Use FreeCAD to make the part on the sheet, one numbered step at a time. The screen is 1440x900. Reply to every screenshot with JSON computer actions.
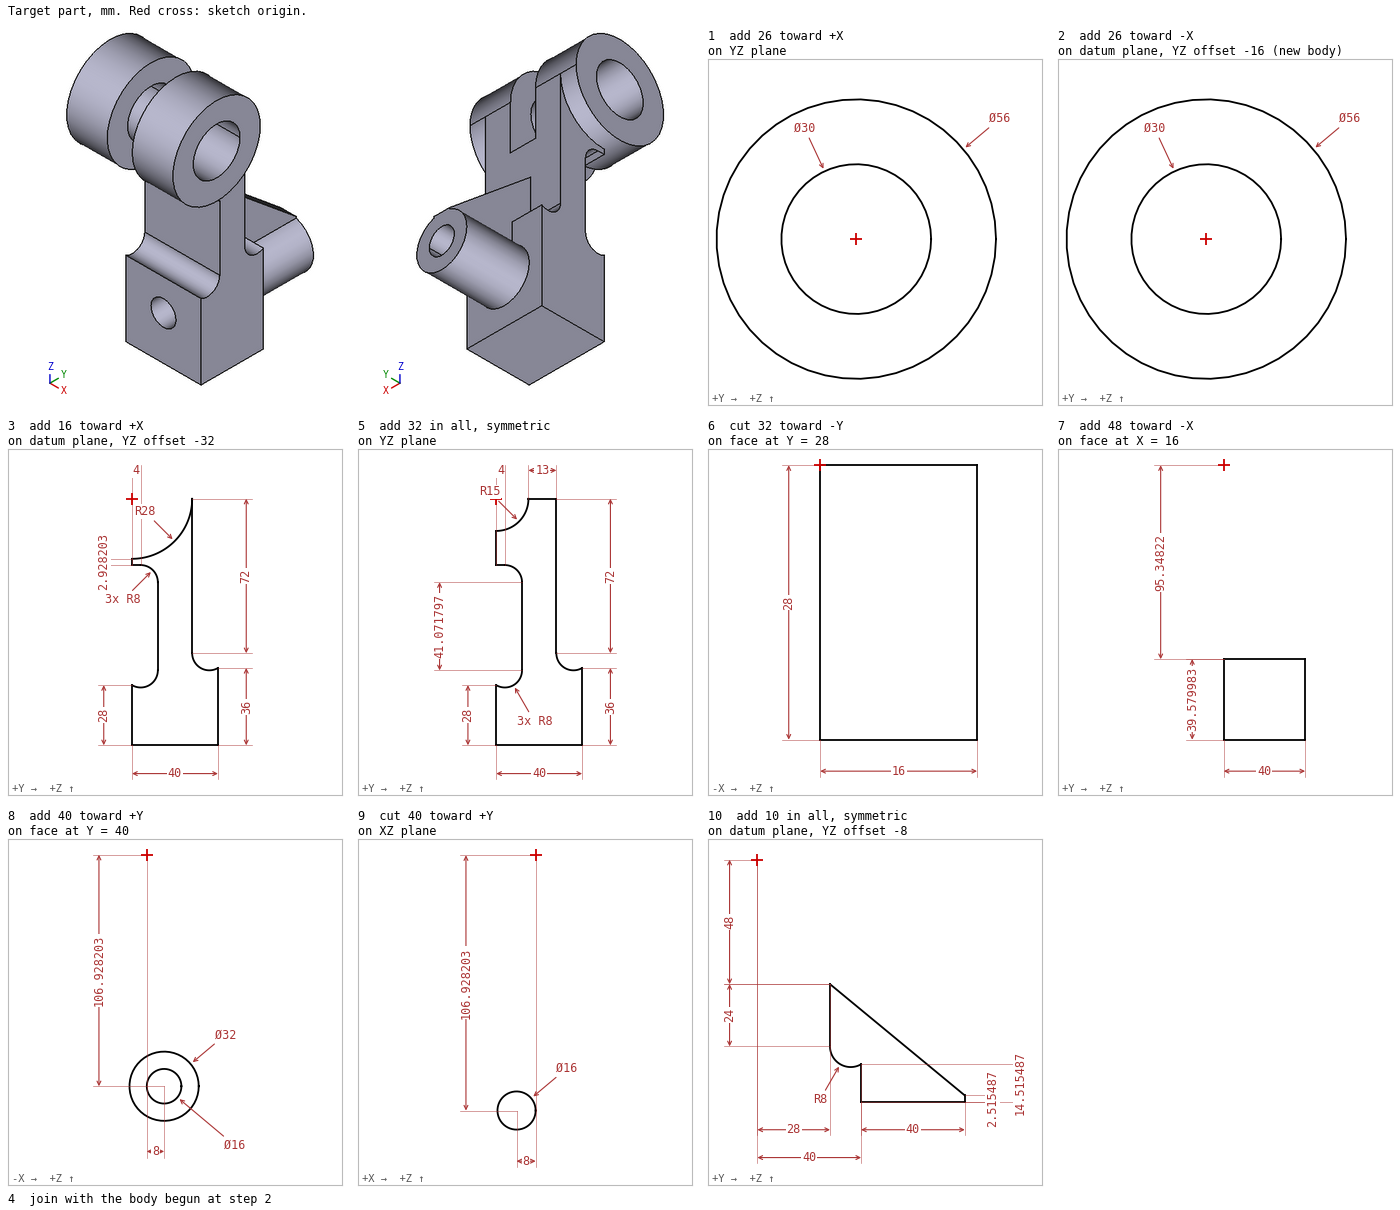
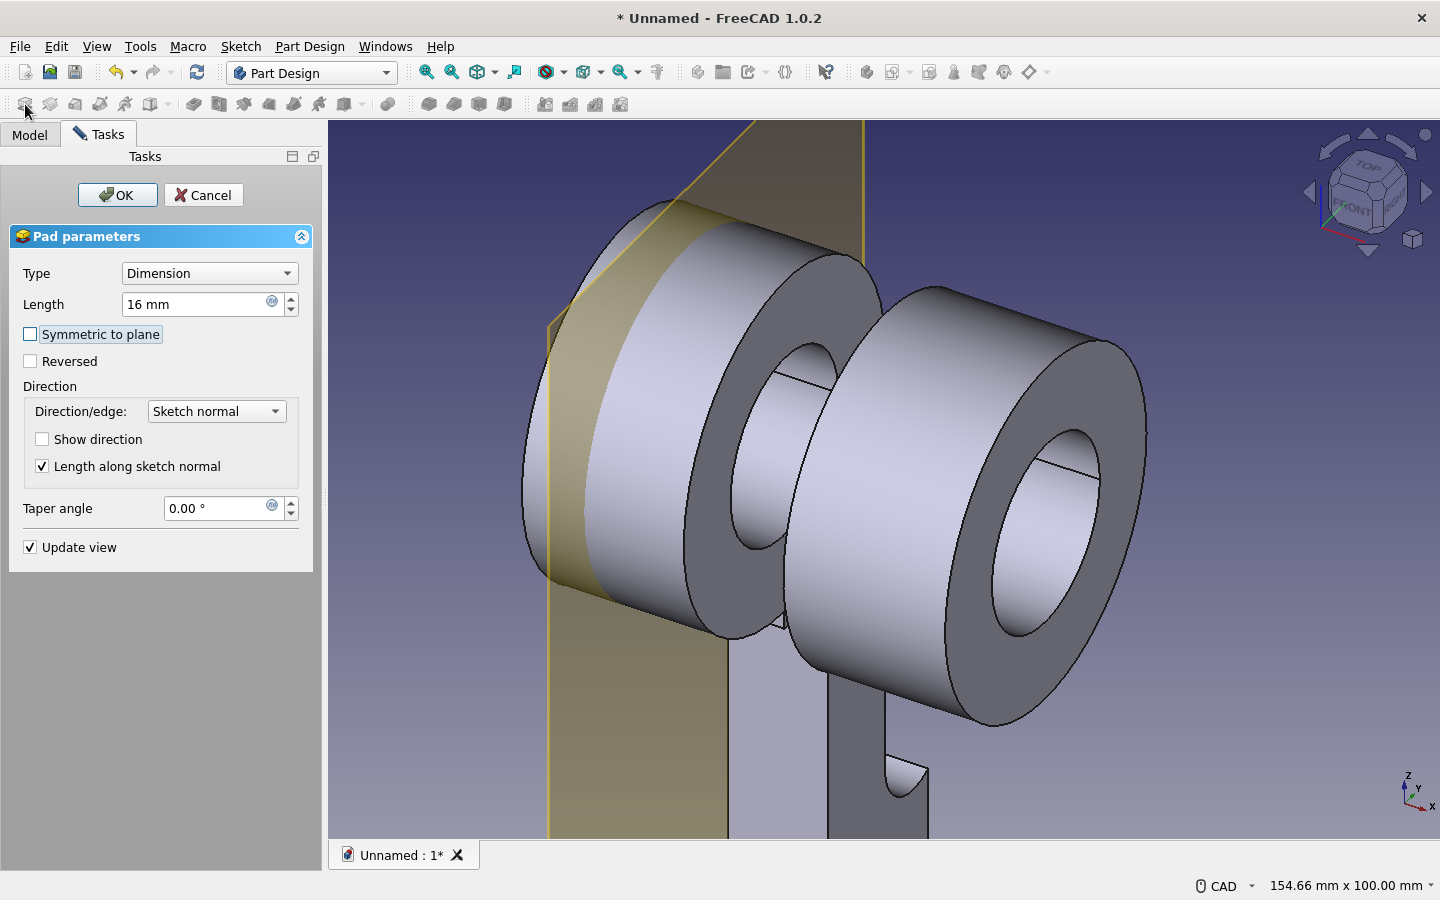
{"action": "left_click", "coordinate": [118, 195]}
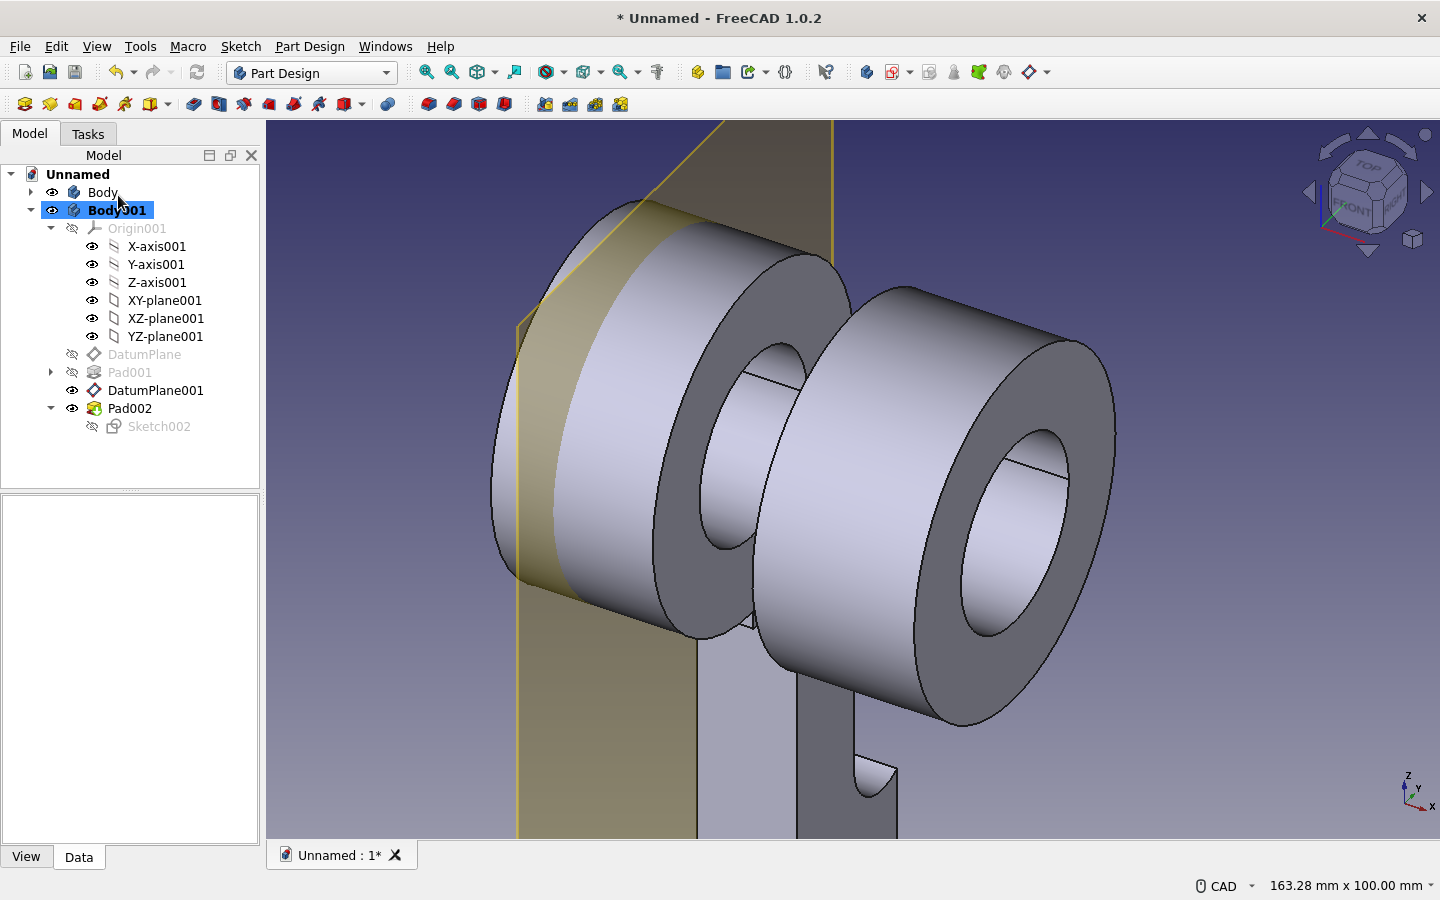
{"action": "left_click", "coordinate": [117, 390]}
{"action": "key", "text": "space"}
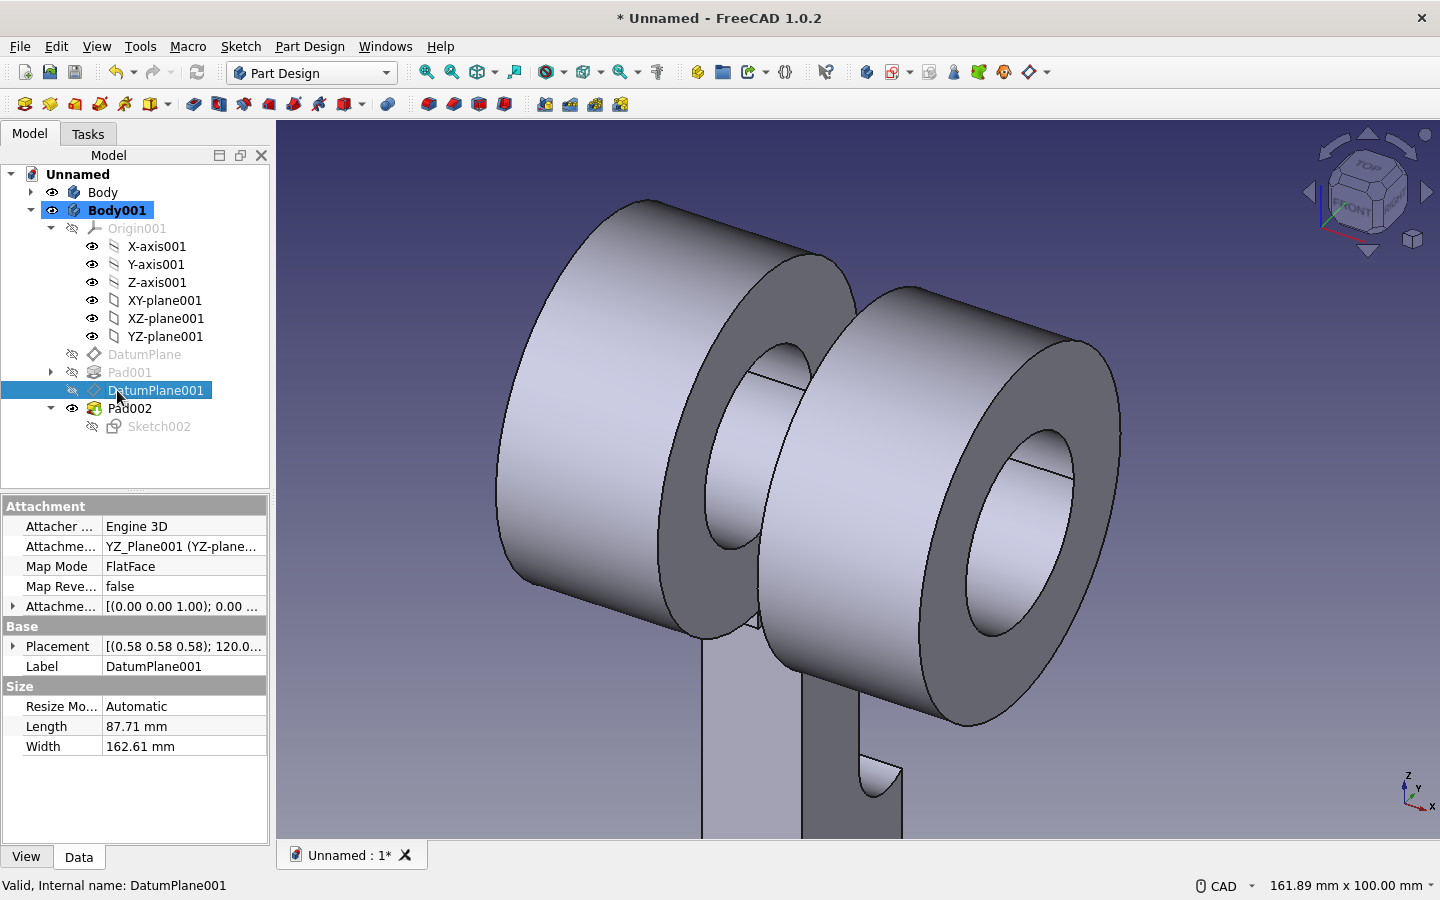
{"action": "key", "text": "v f"}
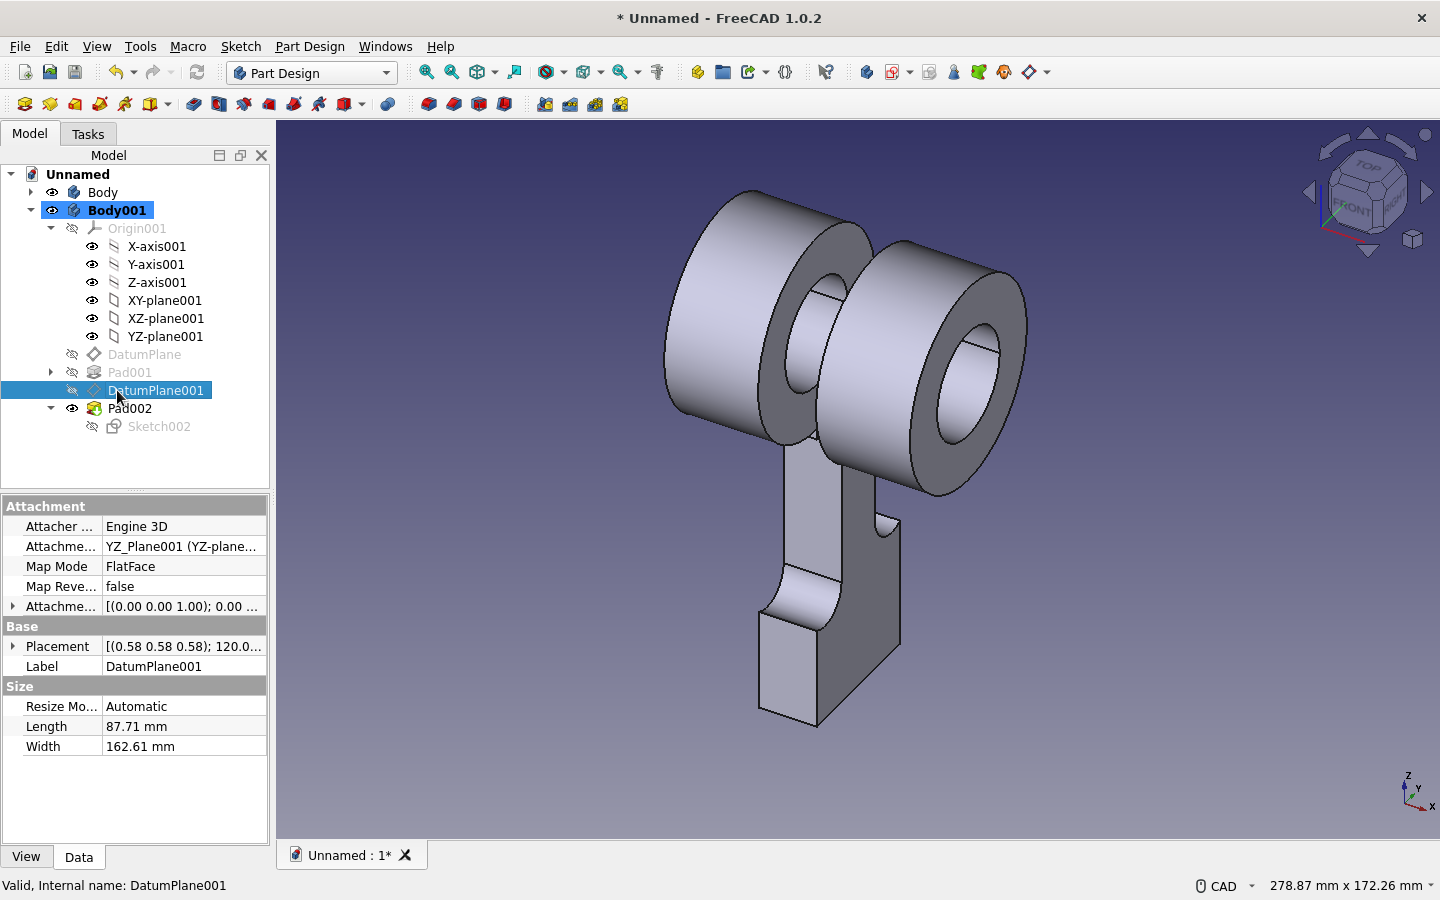
{"action": "double_click", "coordinate": [97, 192]}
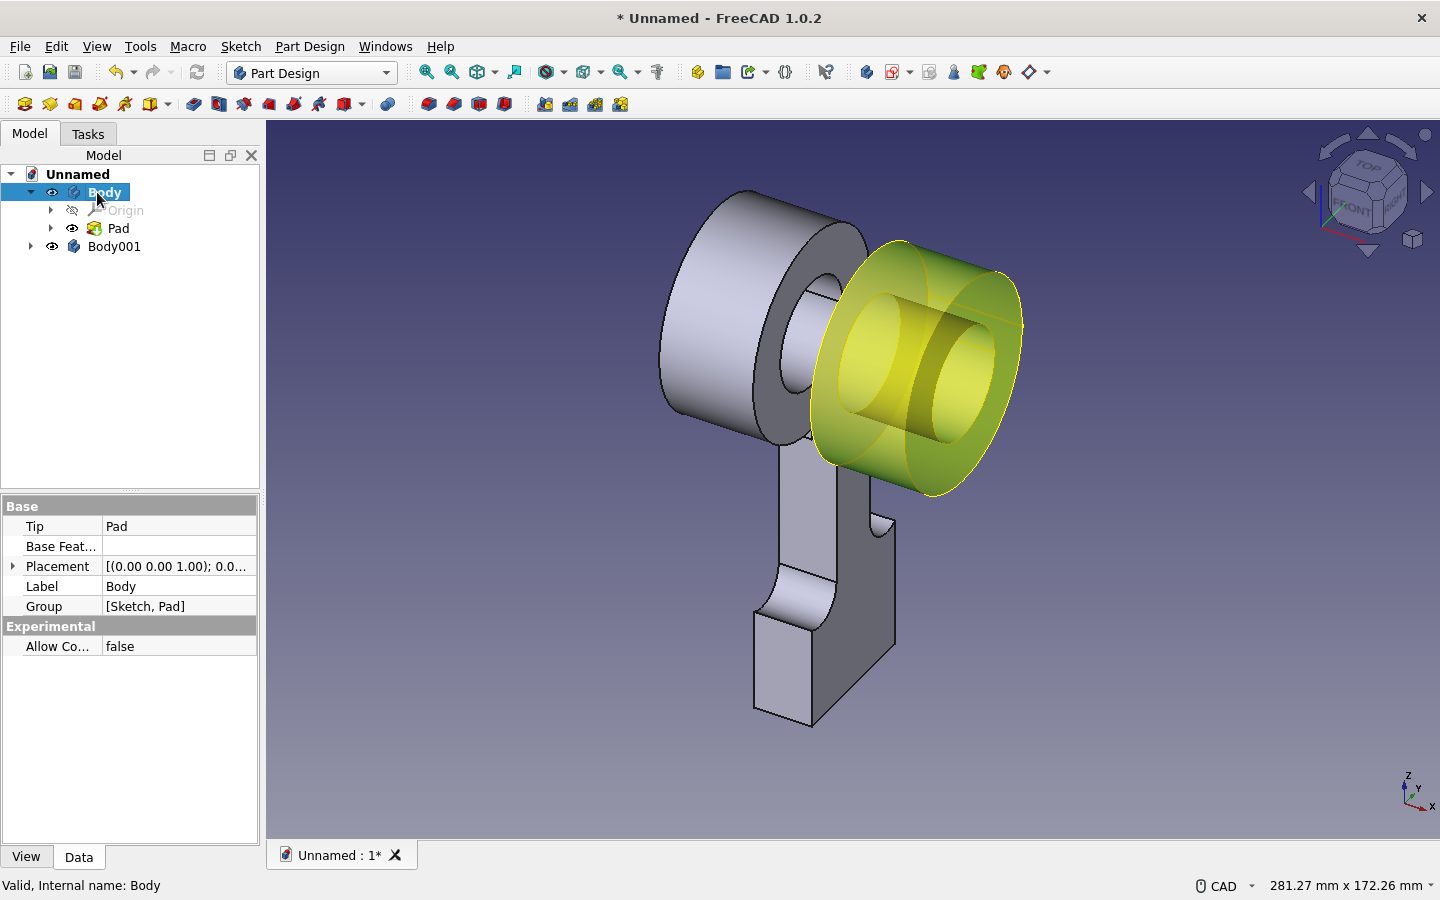
{"action": "left_click", "coordinate": [97, 192]}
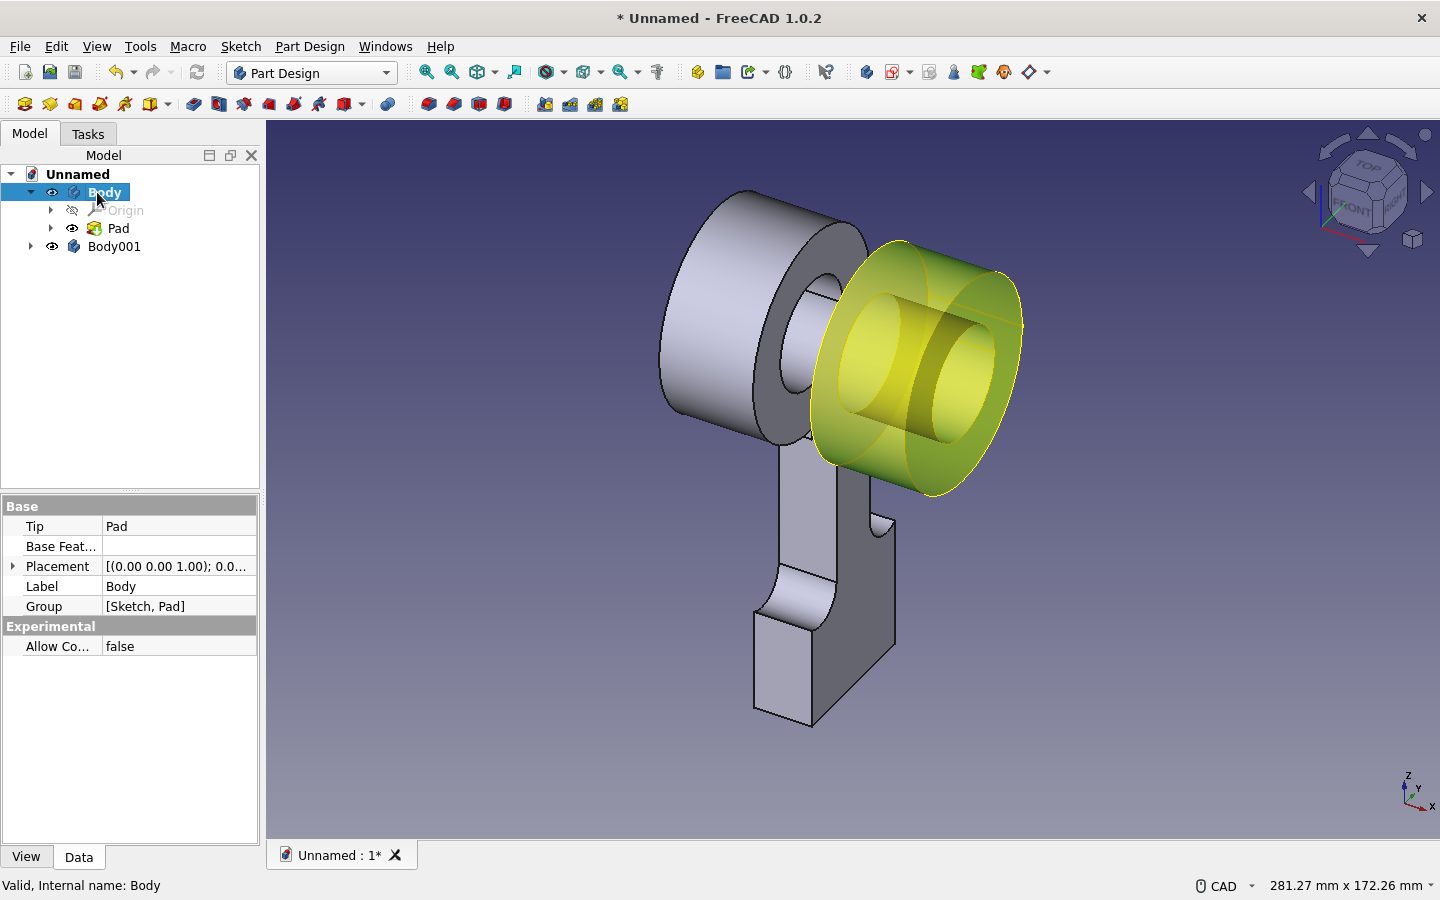
{"action": "left_click", "coordinate": [148, 646]}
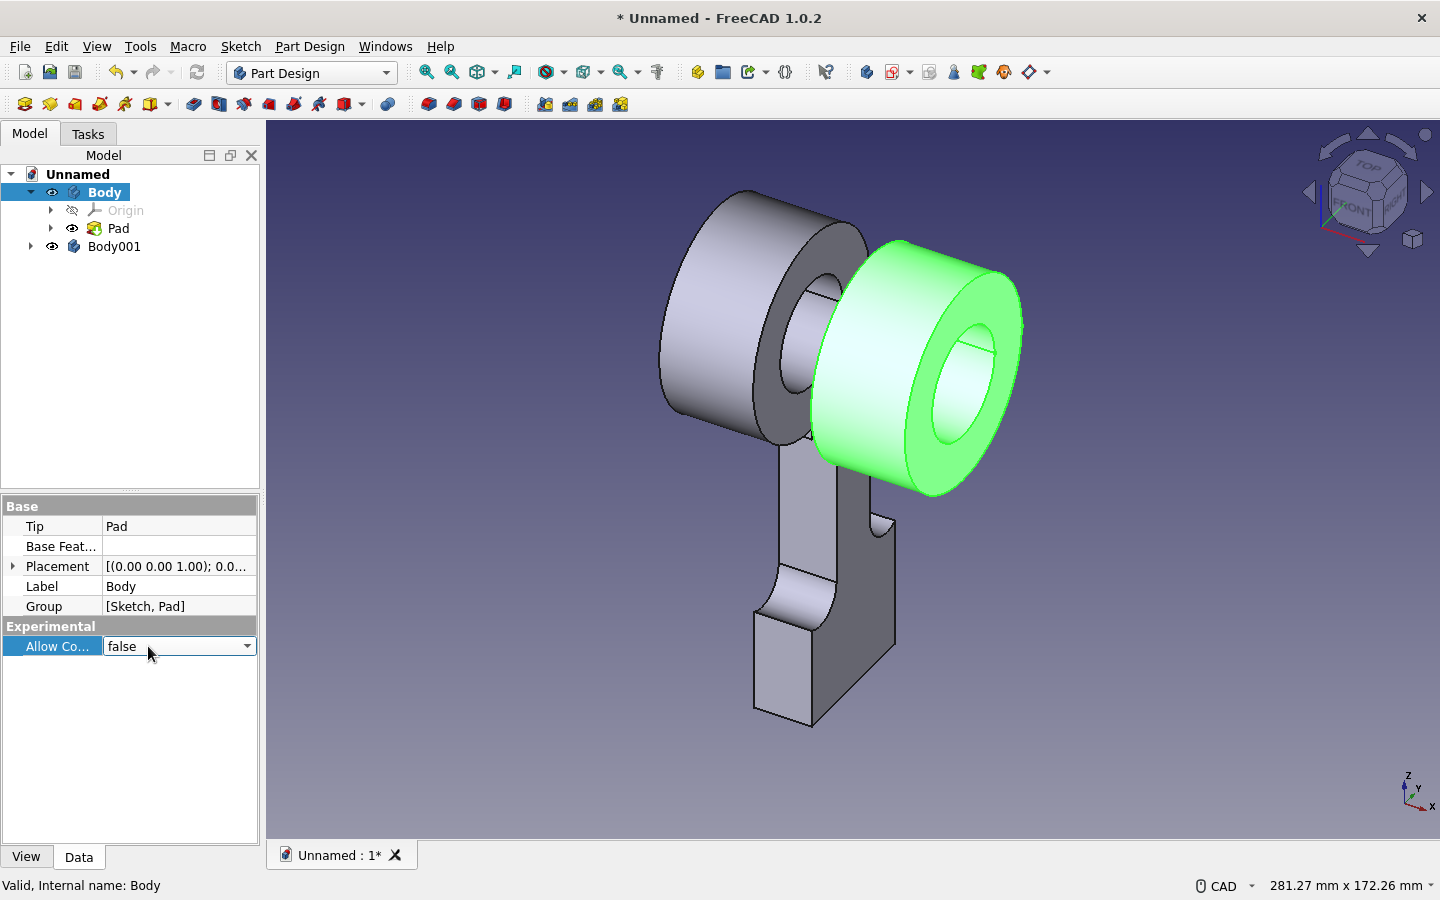
{"action": "left_click", "coordinate": [148, 646]}